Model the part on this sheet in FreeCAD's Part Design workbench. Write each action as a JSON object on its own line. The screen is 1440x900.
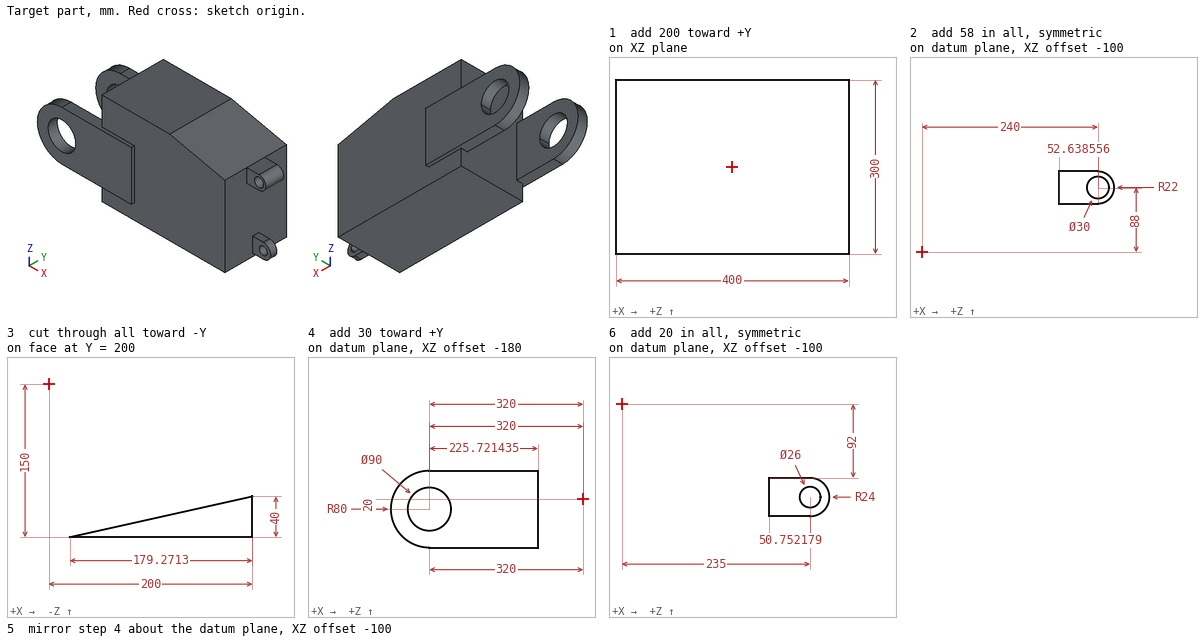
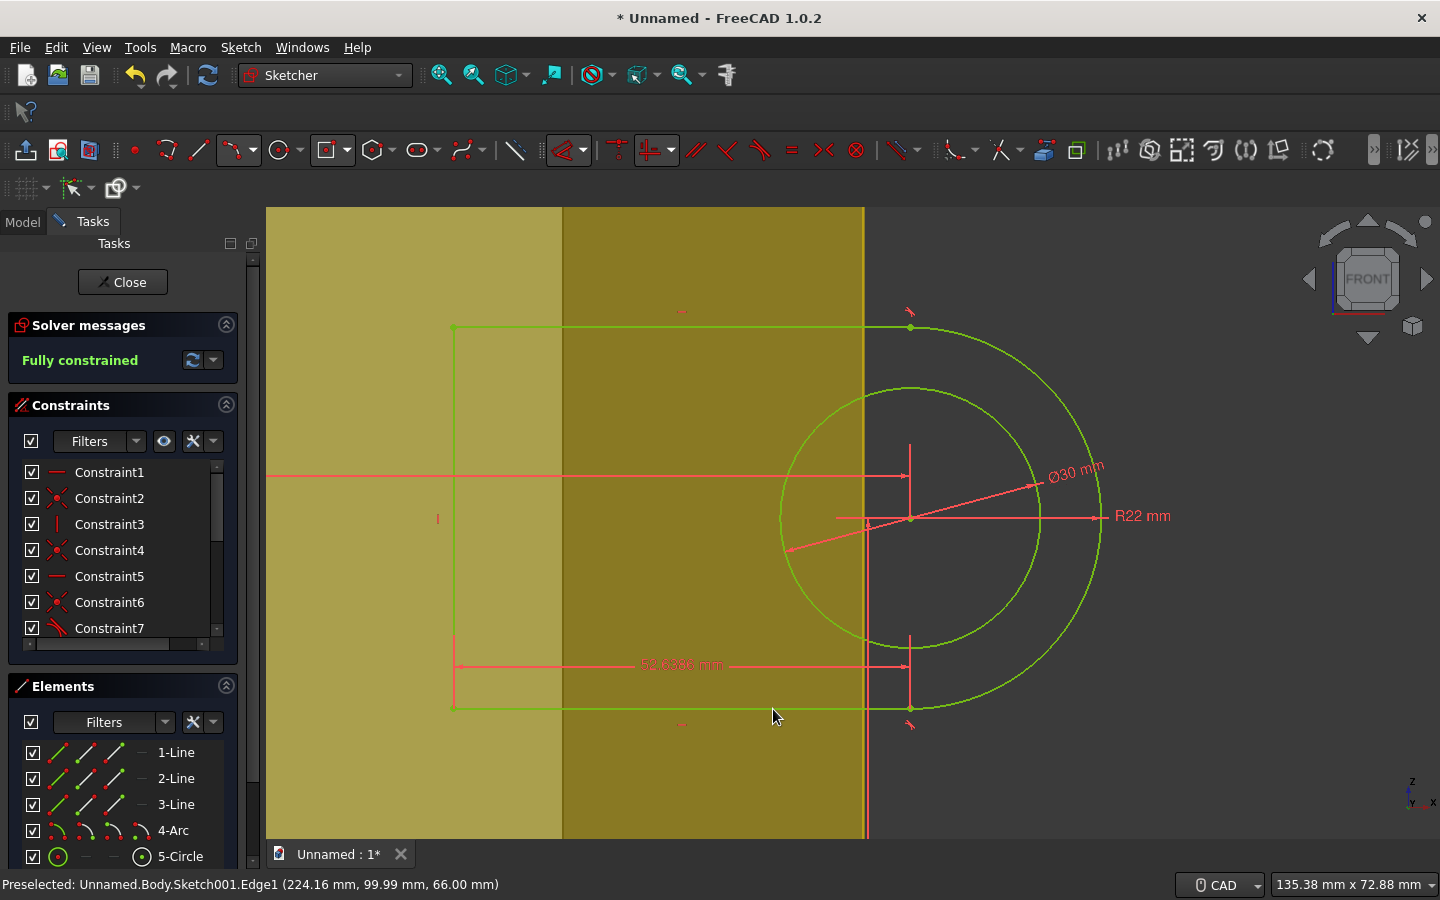
{"action": "left_click", "coordinate": [123, 282]}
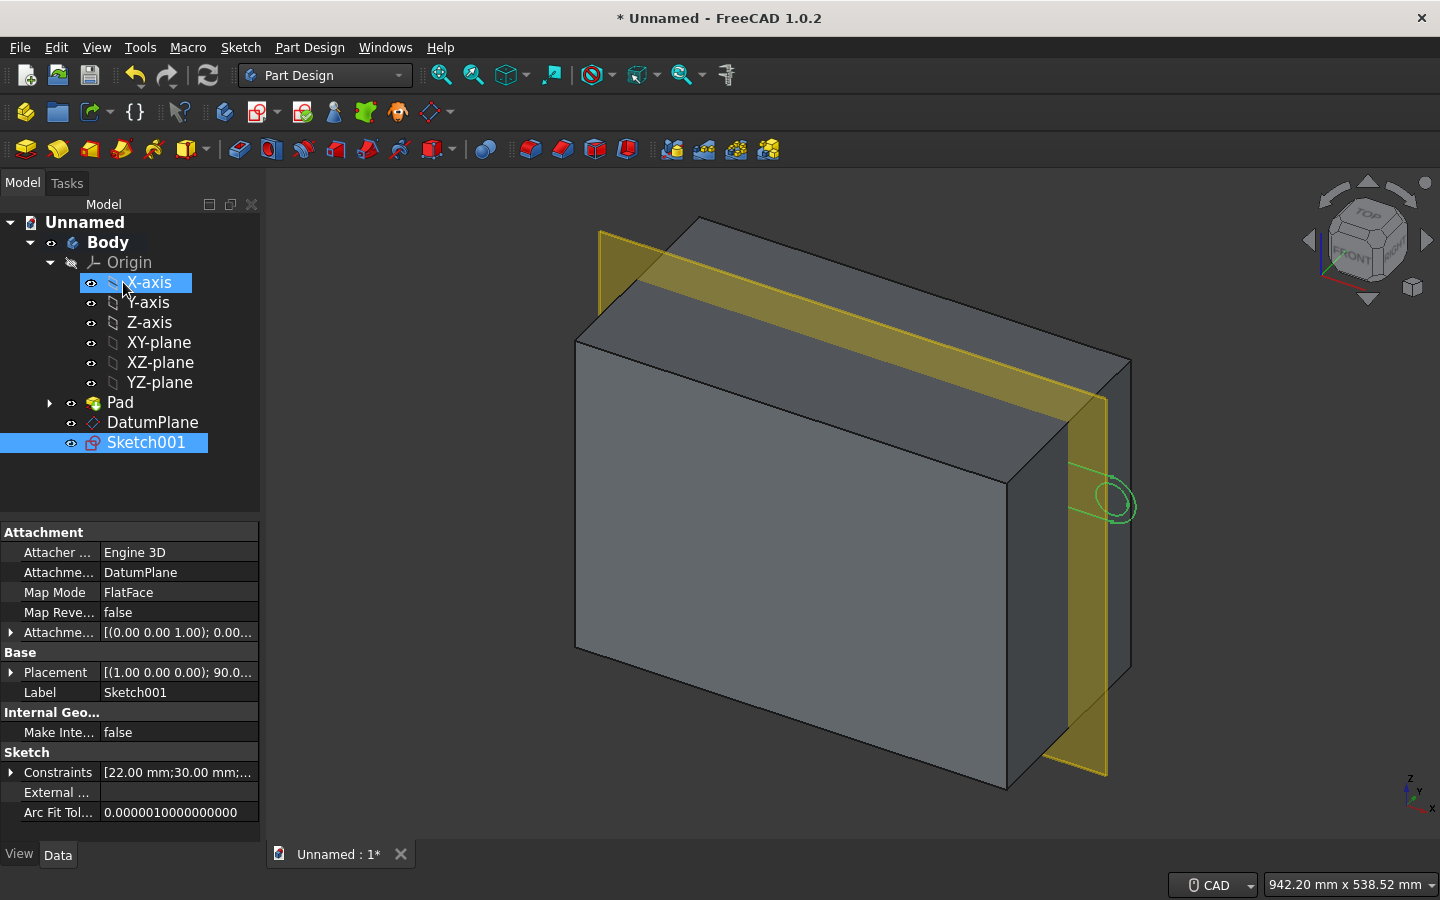
{"action": "left_click", "coordinate": [26, 150]}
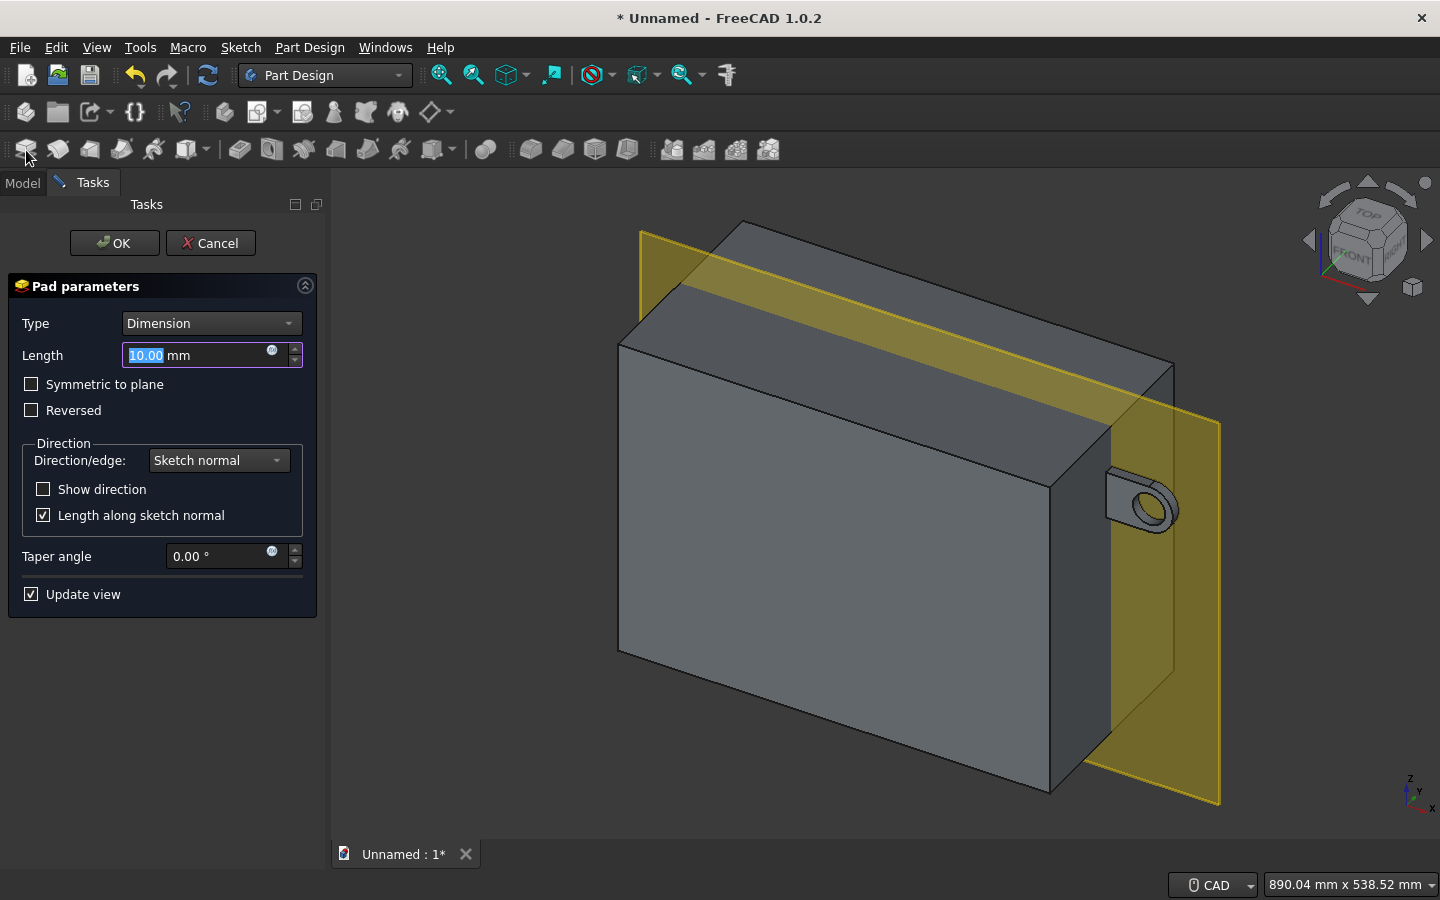
{"action": "type", "text": "58"}
{"action": "key", "text": "Tab"}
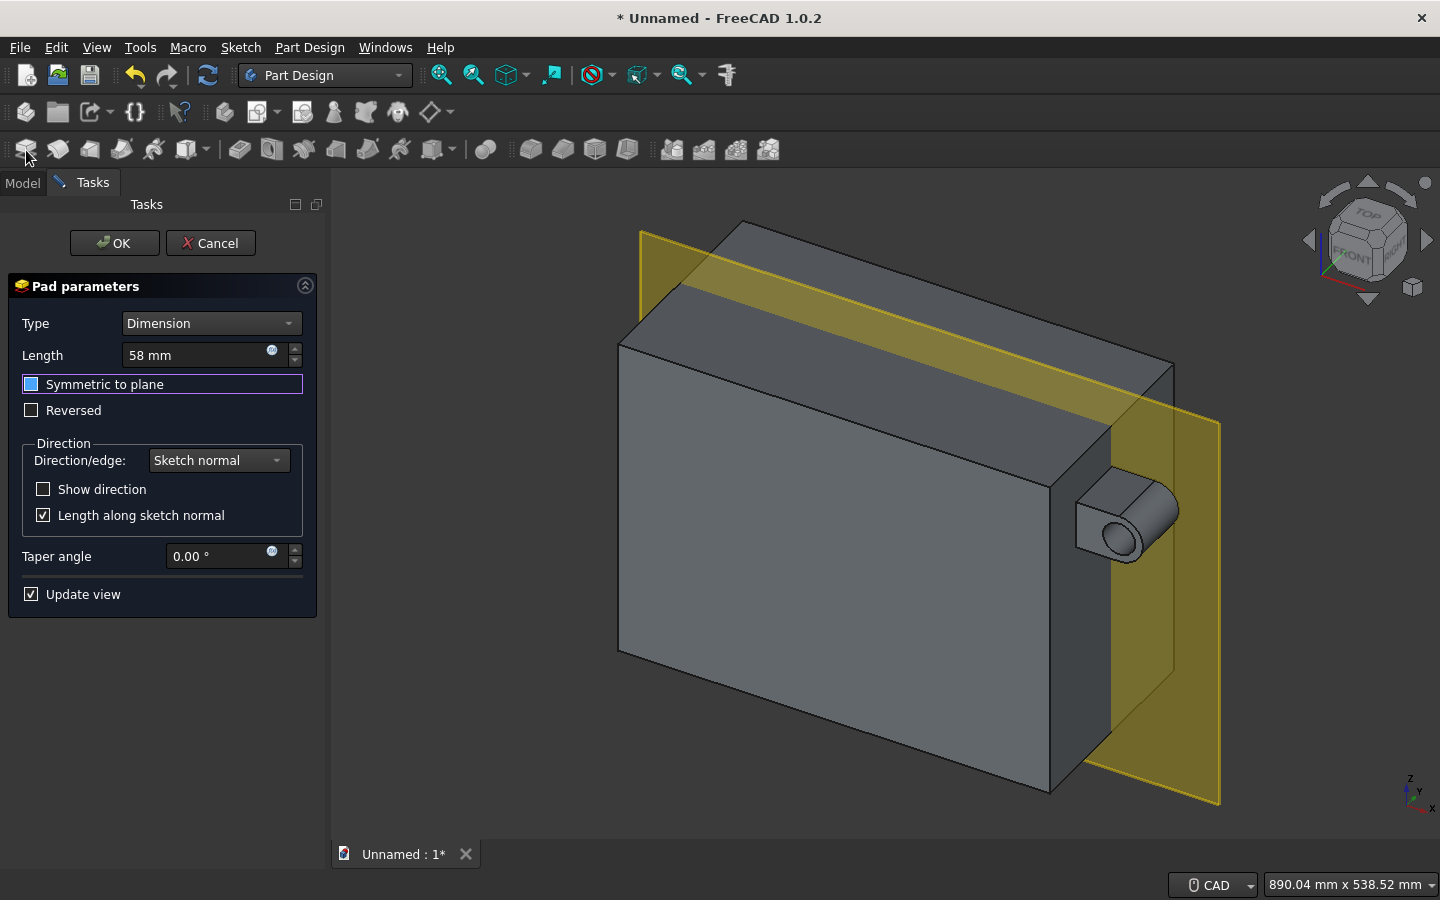
{"action": "left_click", "coordinate": [30, 384]}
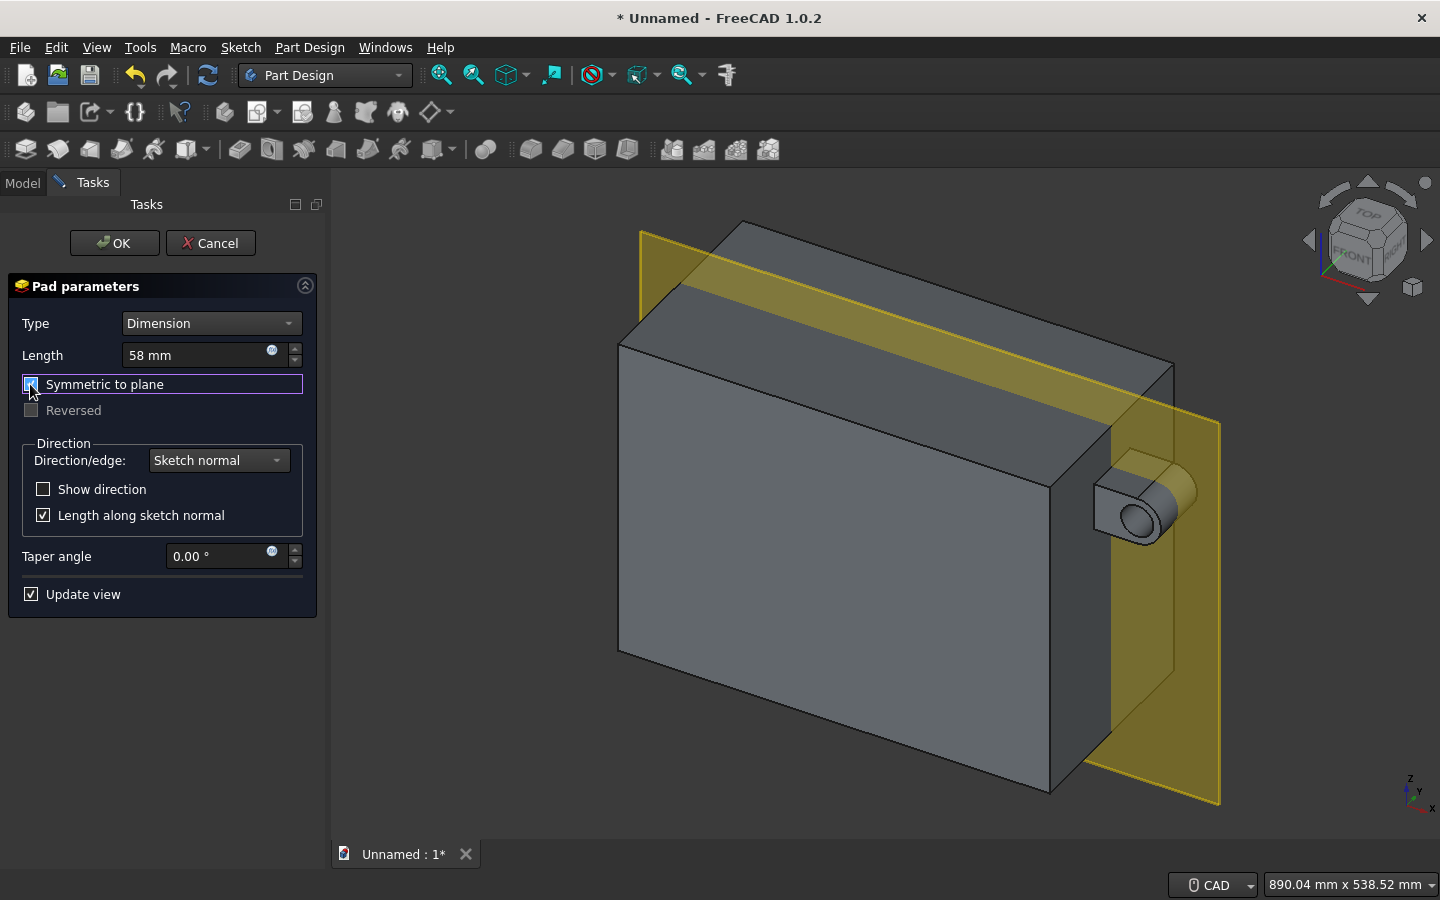
{"action": "left_click", "coordinate": [115, 243]}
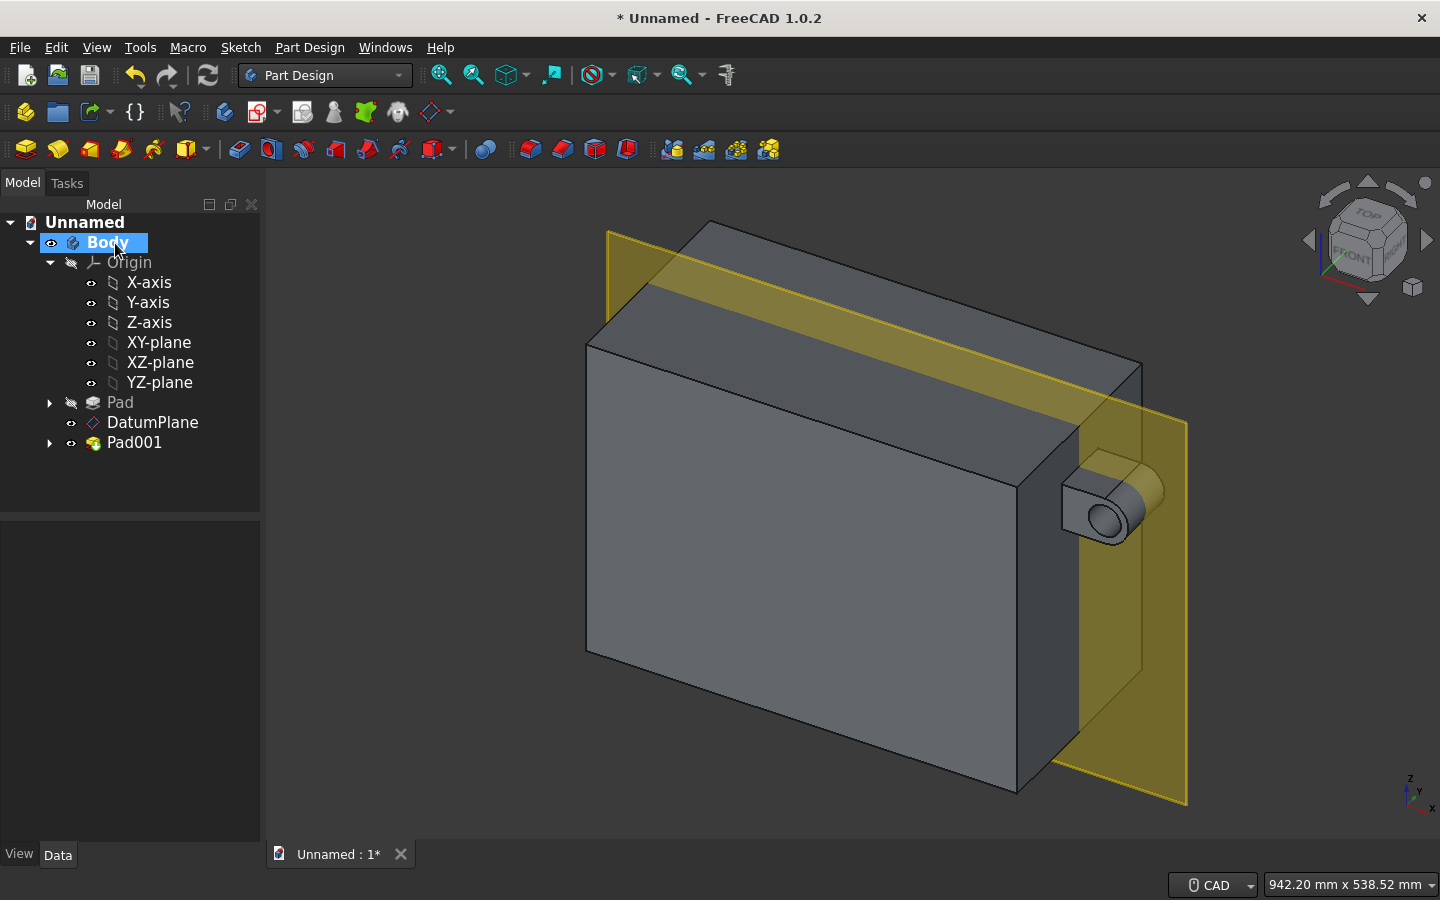
{"action": "left_click", "coordinate": [116, 423]}
{"action": "key", "text": "space"}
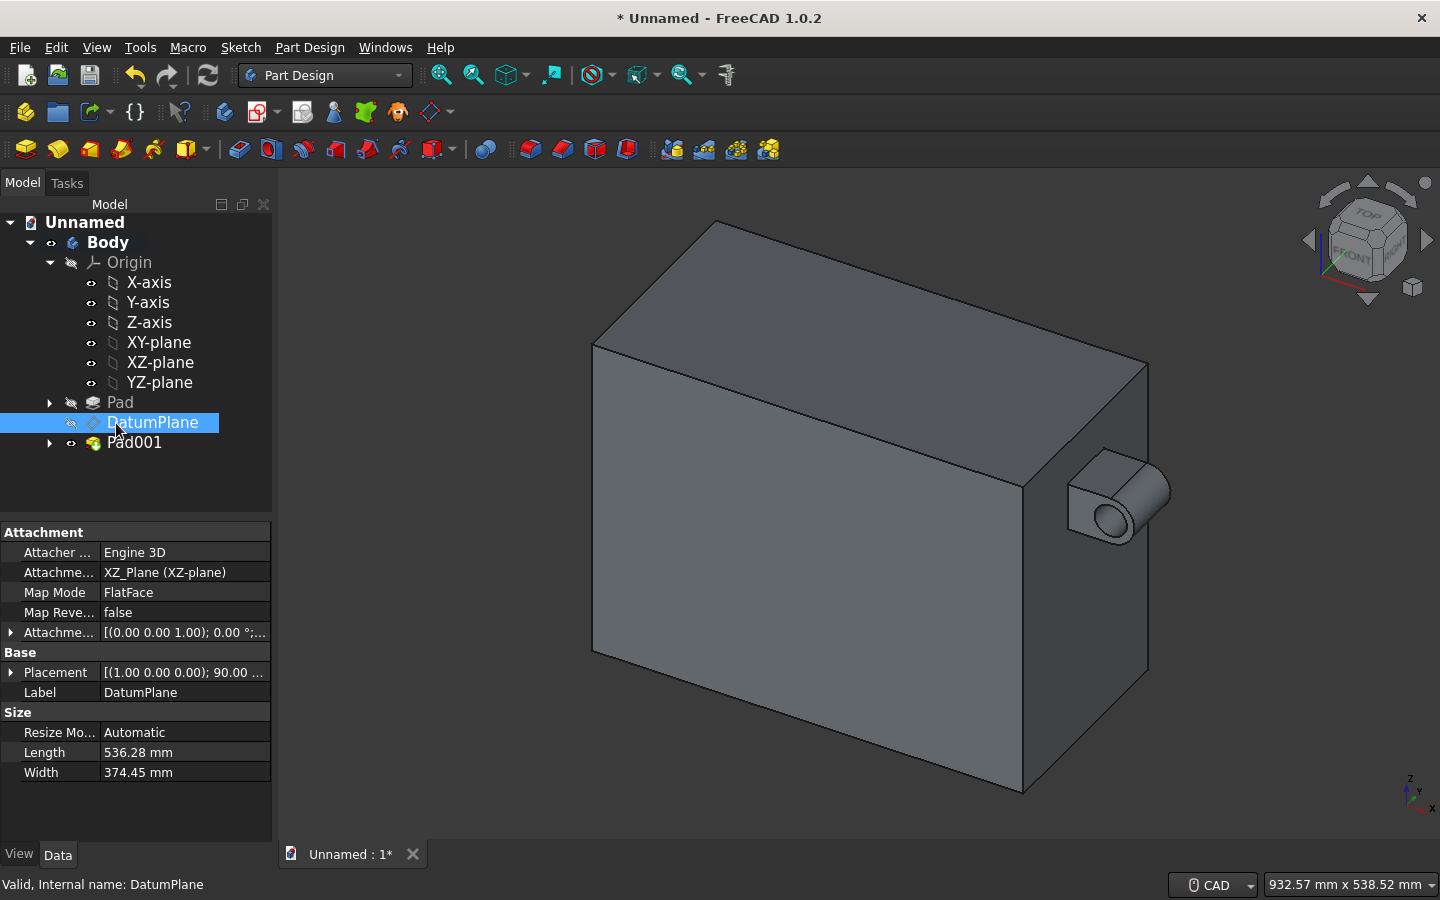
{"action": "key", "text": "4"}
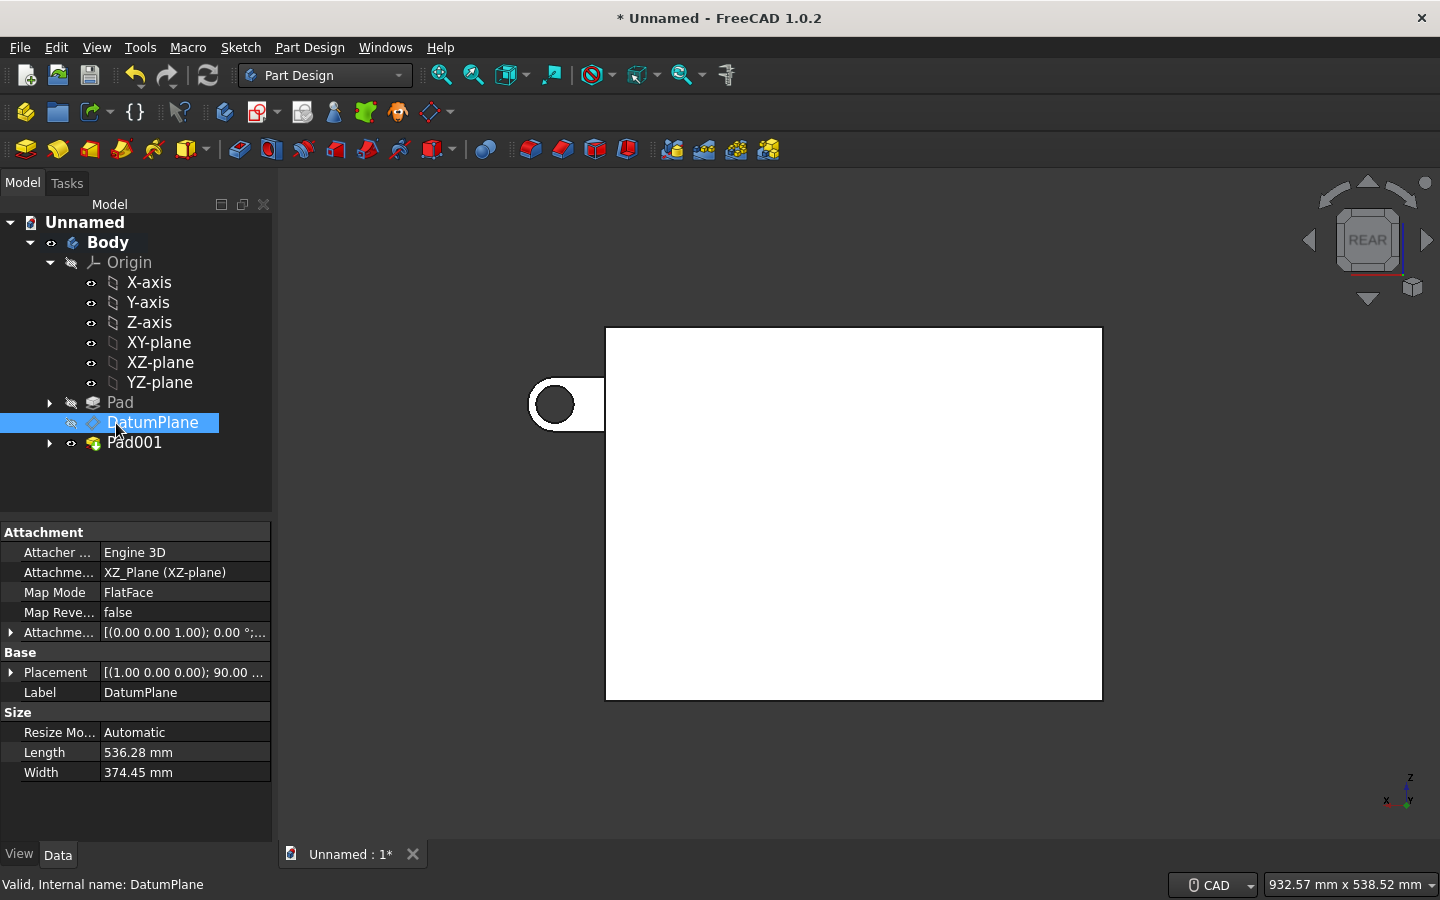
{"action": "left_click", "coordinate": [854, 513]}